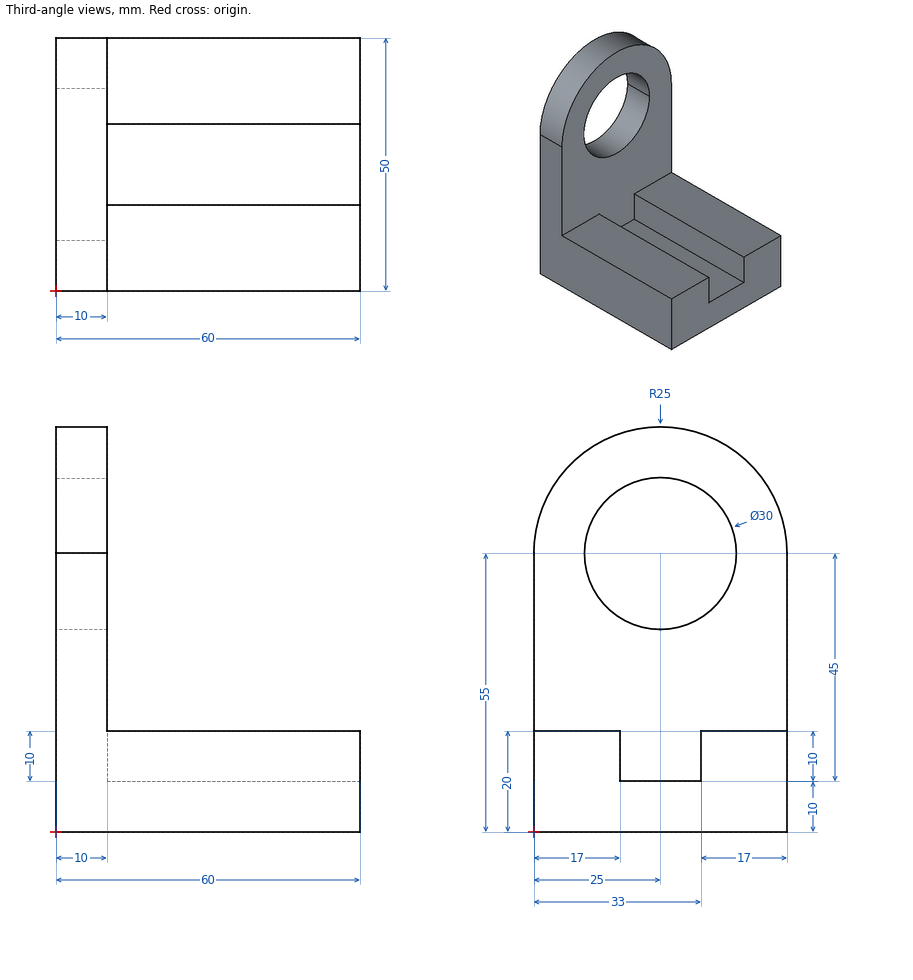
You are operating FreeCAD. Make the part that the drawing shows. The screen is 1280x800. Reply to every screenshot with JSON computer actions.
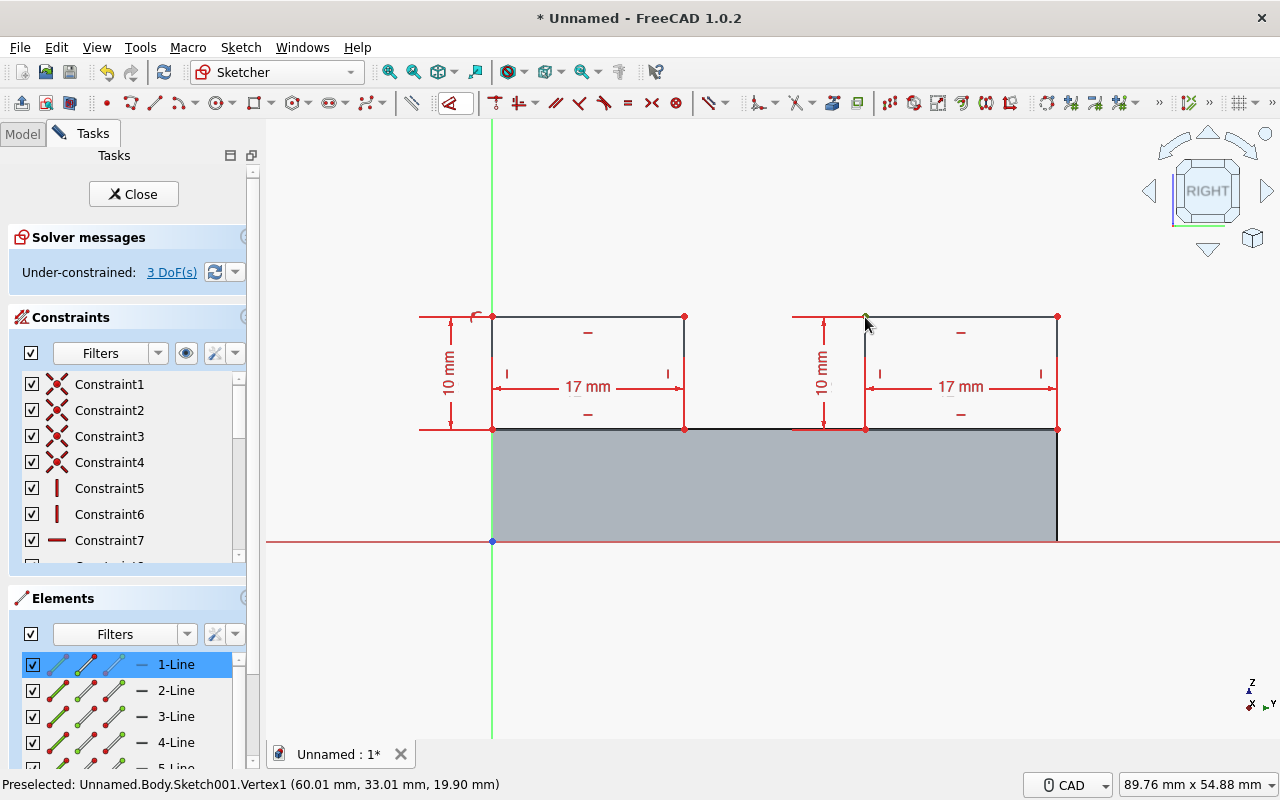
{"action": "key", "text": "l"}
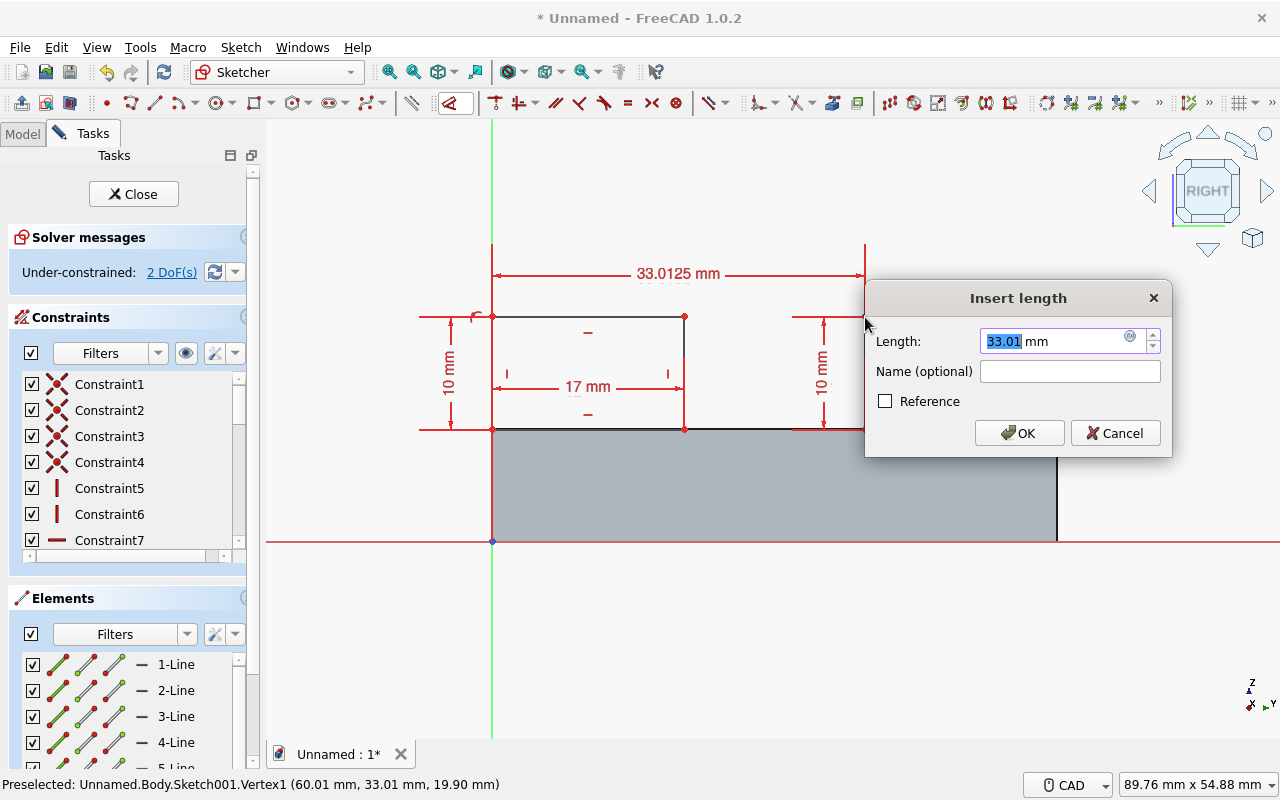
{"action": "type", "text": "33"}
{"action": "key", "text": "Return"}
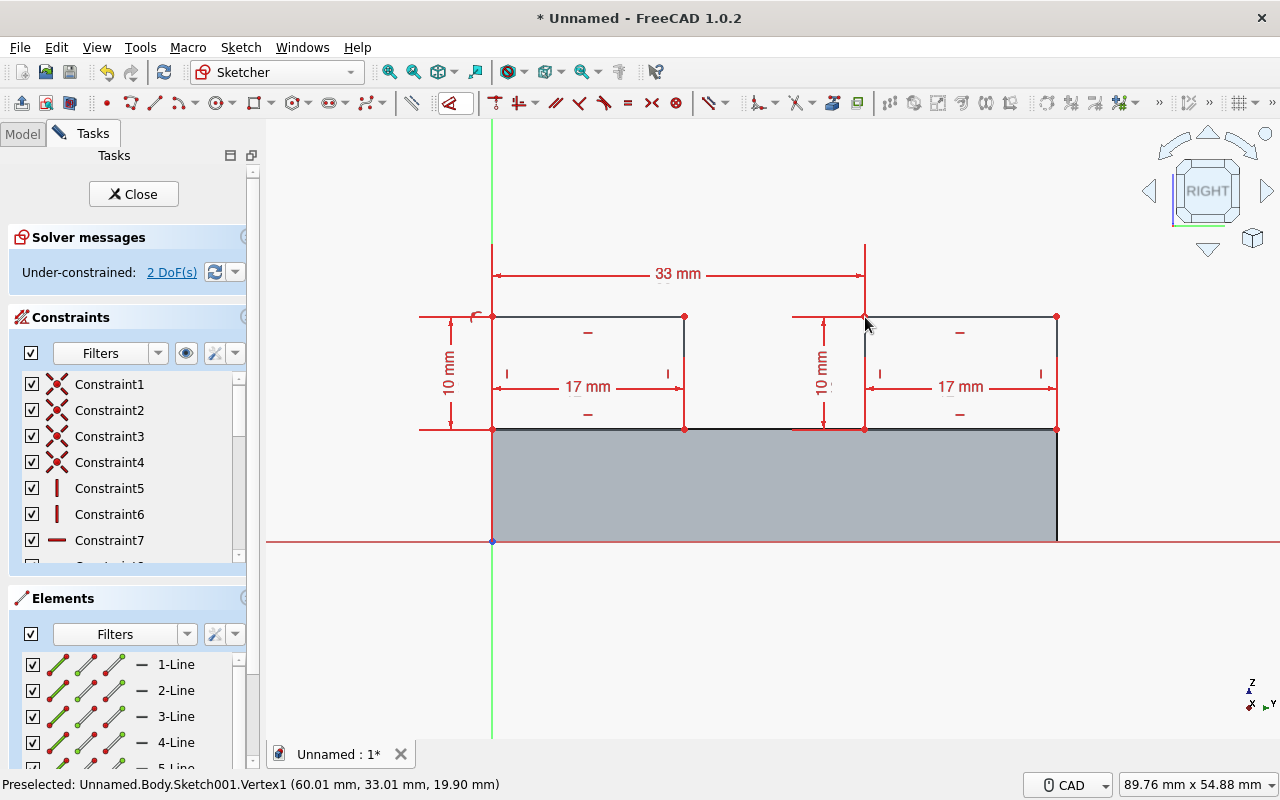
{"action": "left_click", "coordinate": [865, 317]}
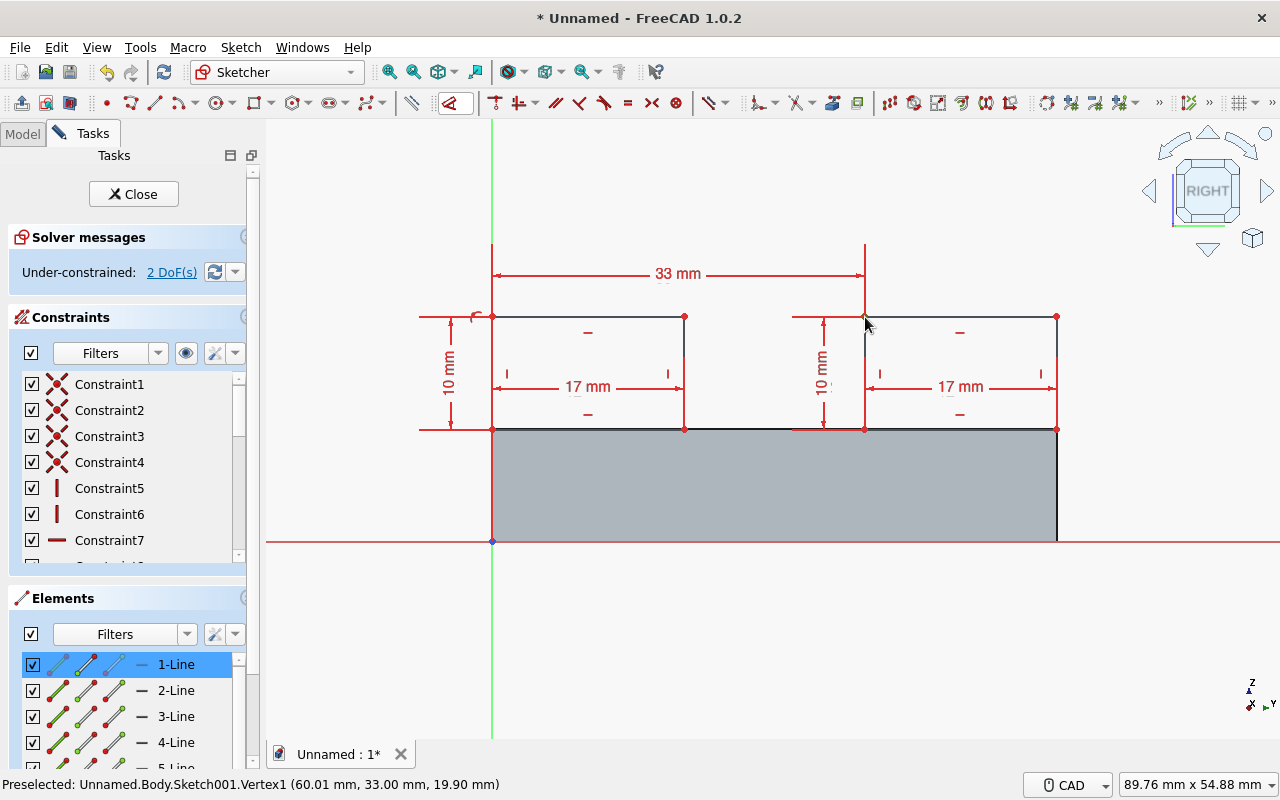
{"action": "key", "text": "i"}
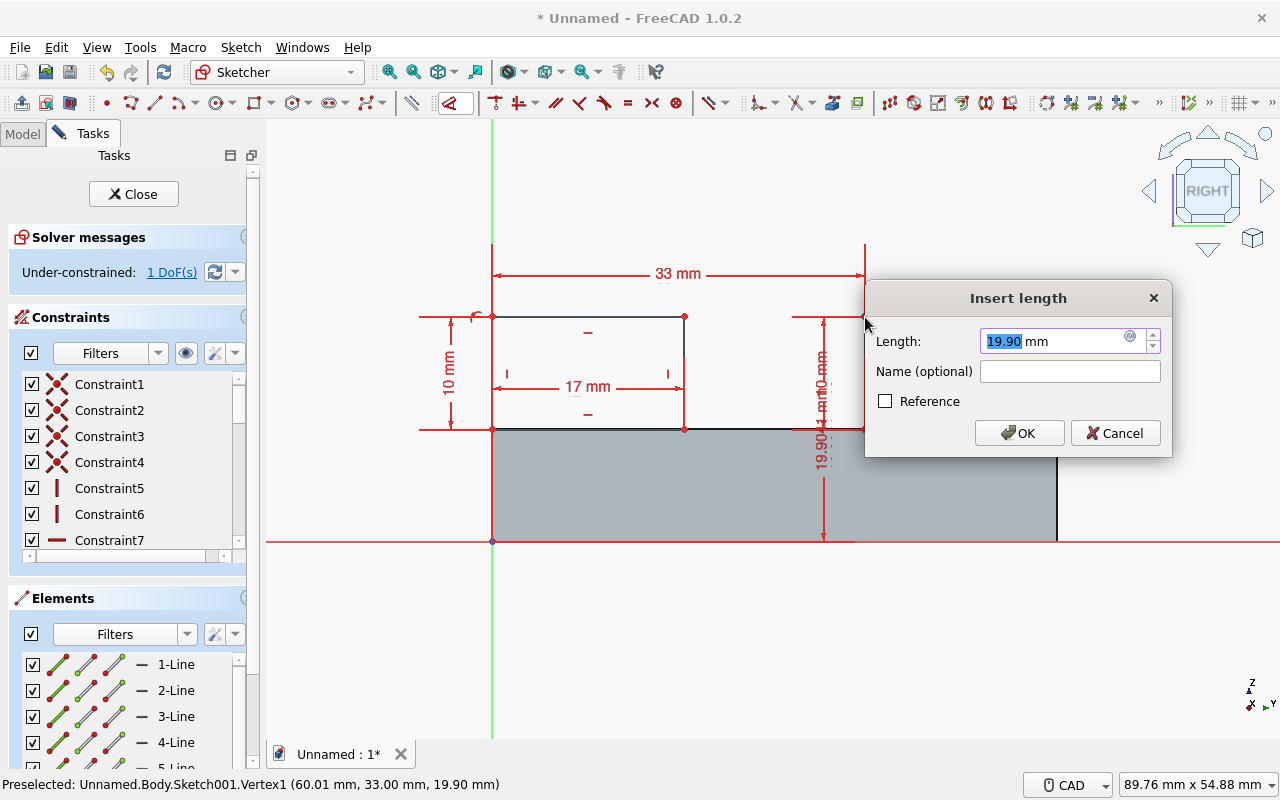
{"action": "type", "text": "20"}
{"action": "key", "text": "Return"}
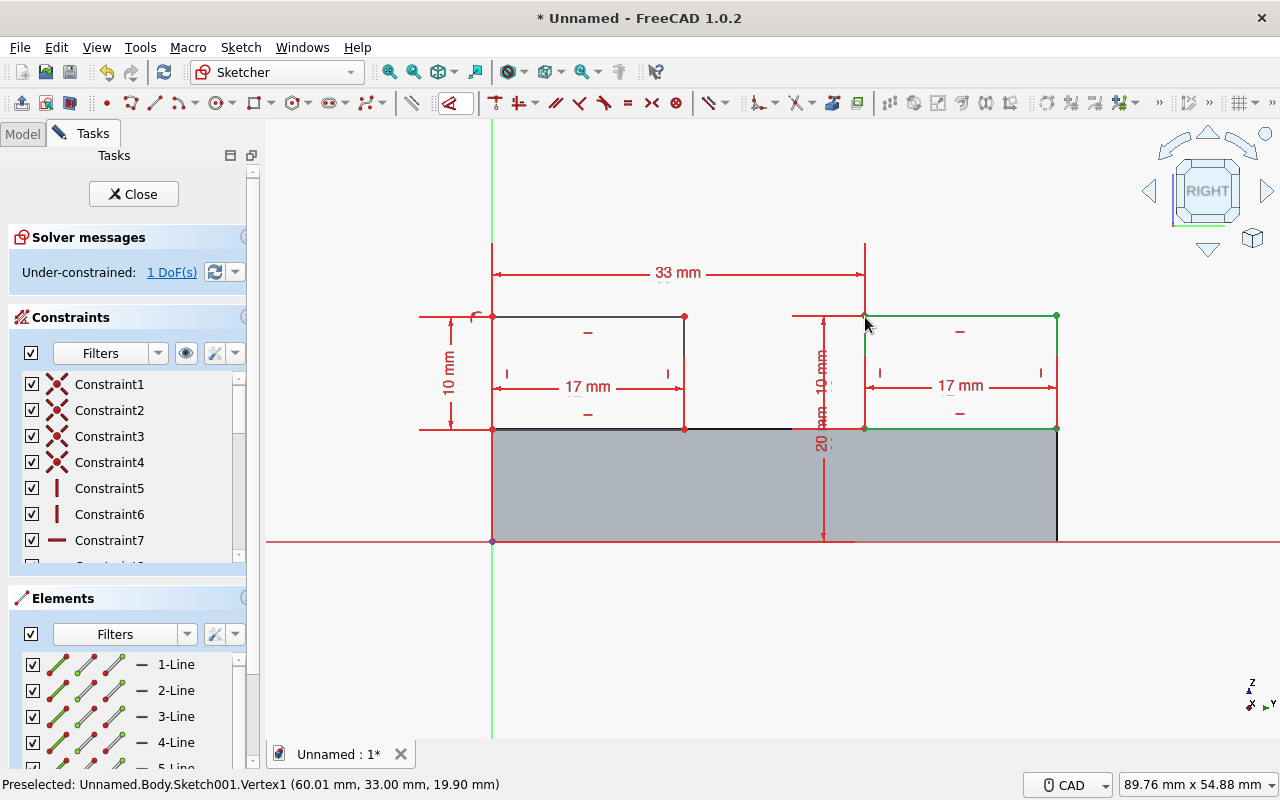
{"action": "left_click", "coordinate": [492, 317]}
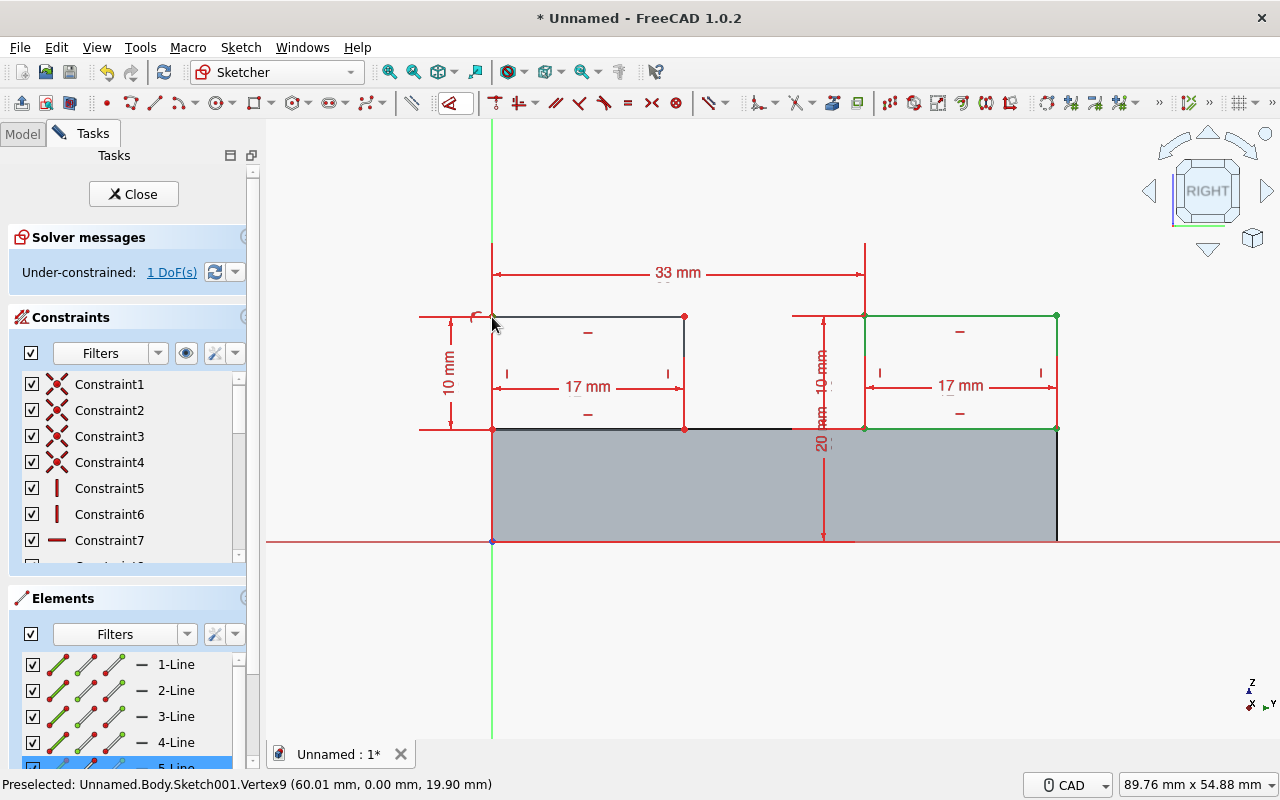
{"action": "key", "text": "i"}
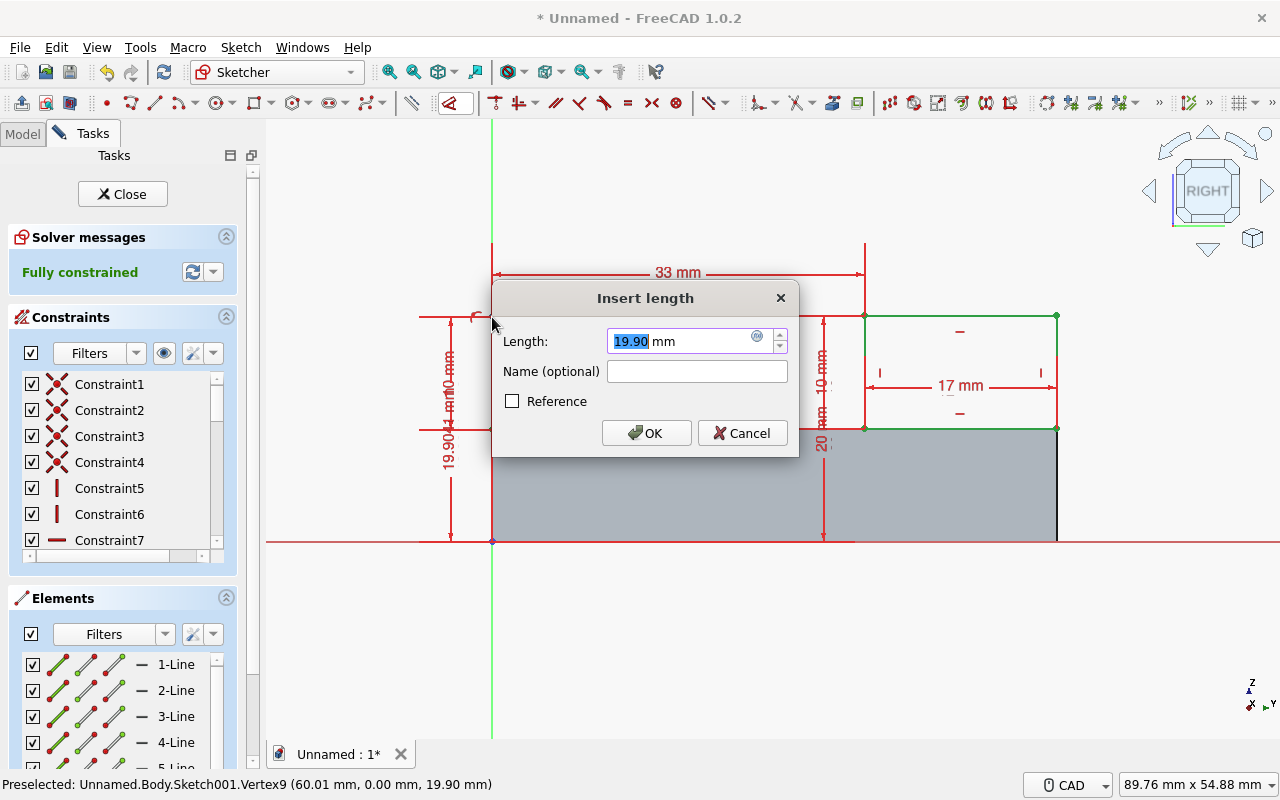
{"action": "type", "text": "20"}
{"action": "key", "text": "Return"}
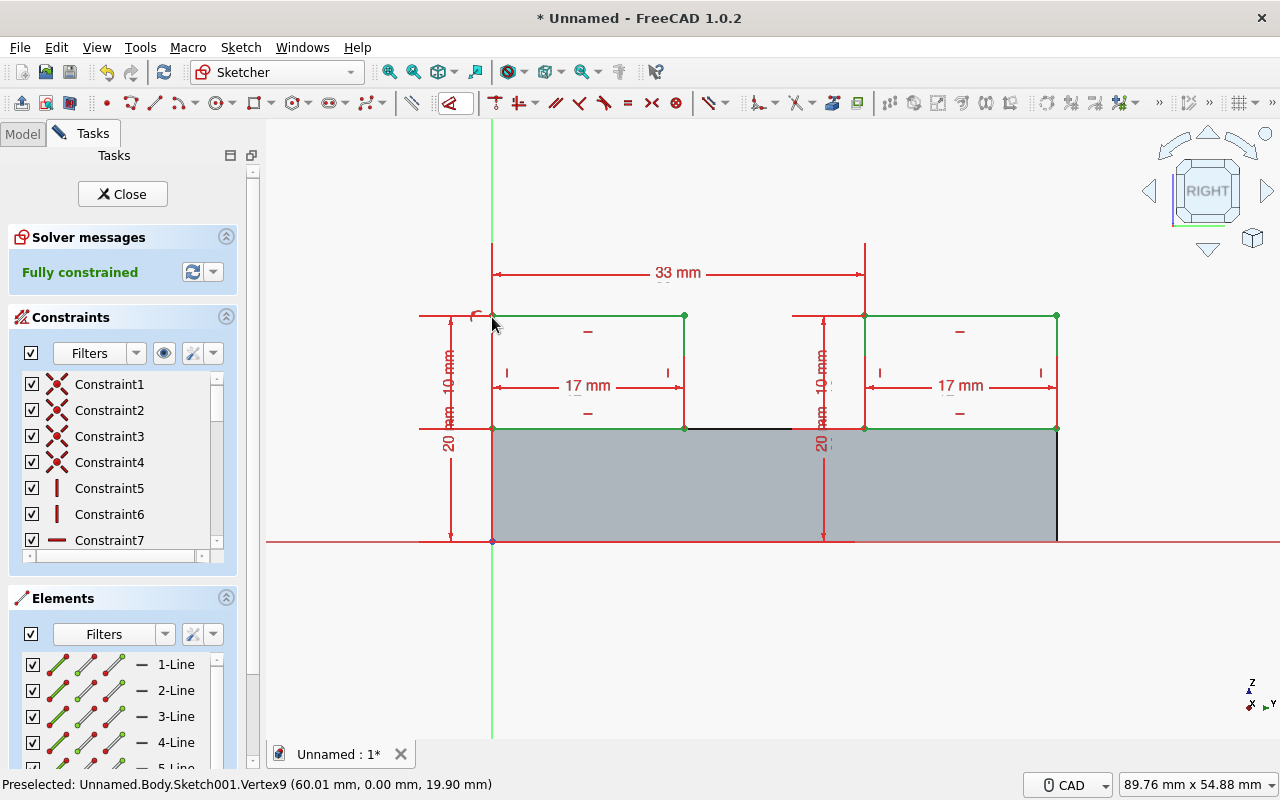
{"action": "left_click", "coordinate": [123, 194]}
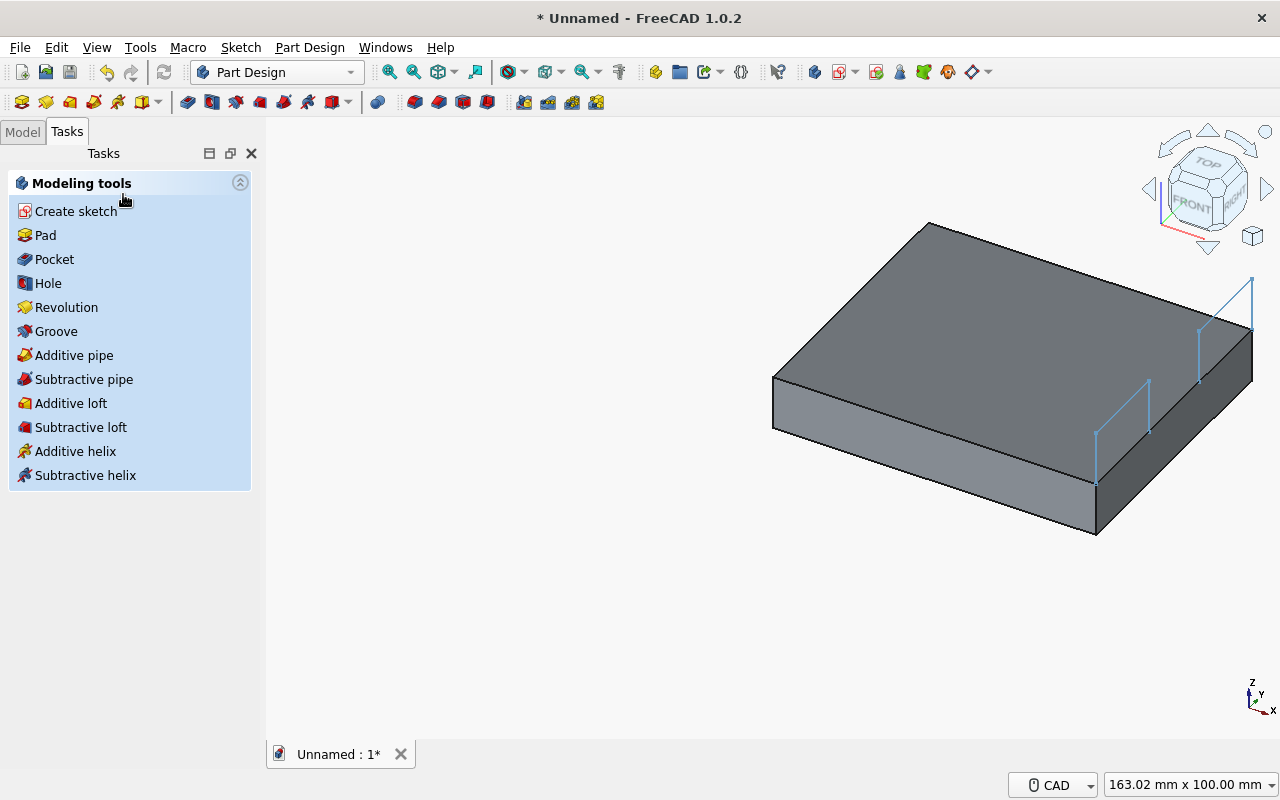
{"action": "left_click", "coordinate": [22, 102]}